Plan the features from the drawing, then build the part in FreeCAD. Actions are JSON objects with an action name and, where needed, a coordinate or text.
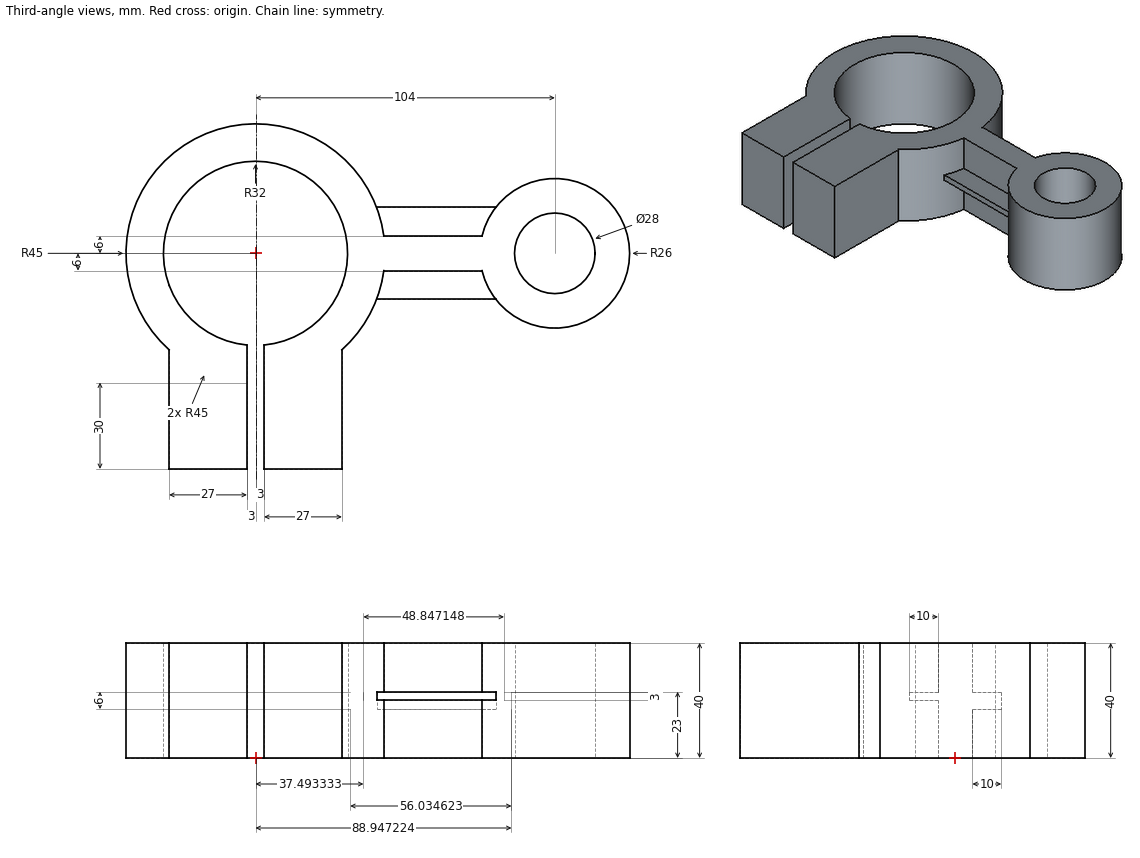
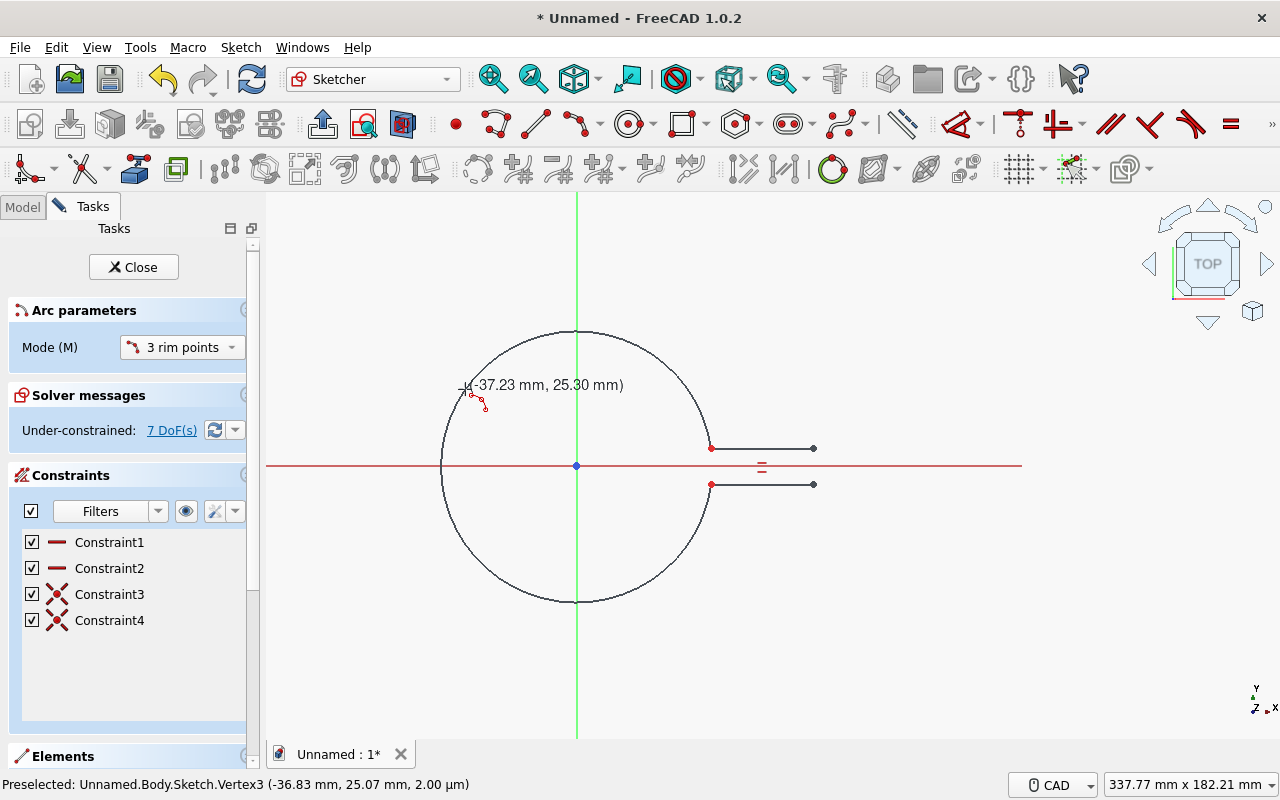
{"action": "left_click", "coordinate": [813, 485]}
{"action": "left_click", "coordinate": [813, 449]}
{"action": "left_click", "coordinate": [954, 509]}
{"action": "key", "text": "Escape"}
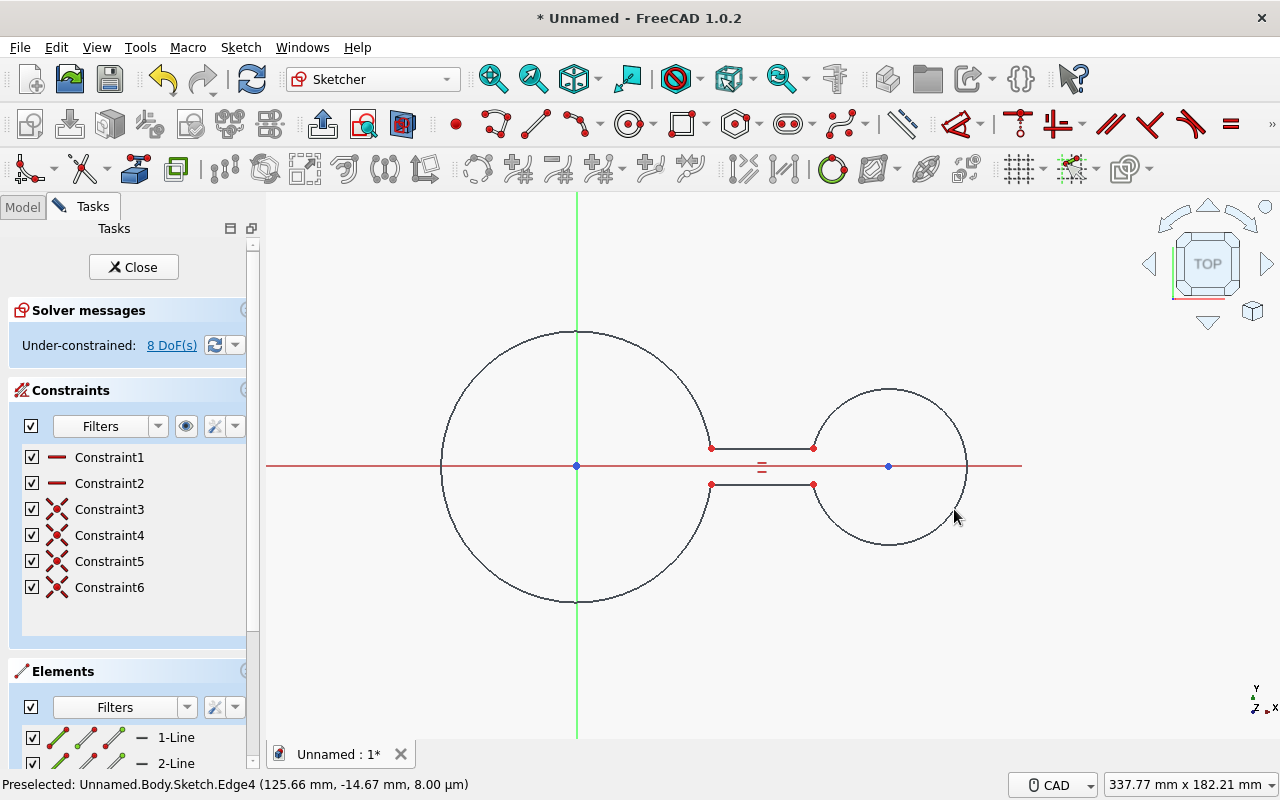
{"action": "left_click_drag", "start_coordinate": [567, 456], "coordinate": [587, 477]}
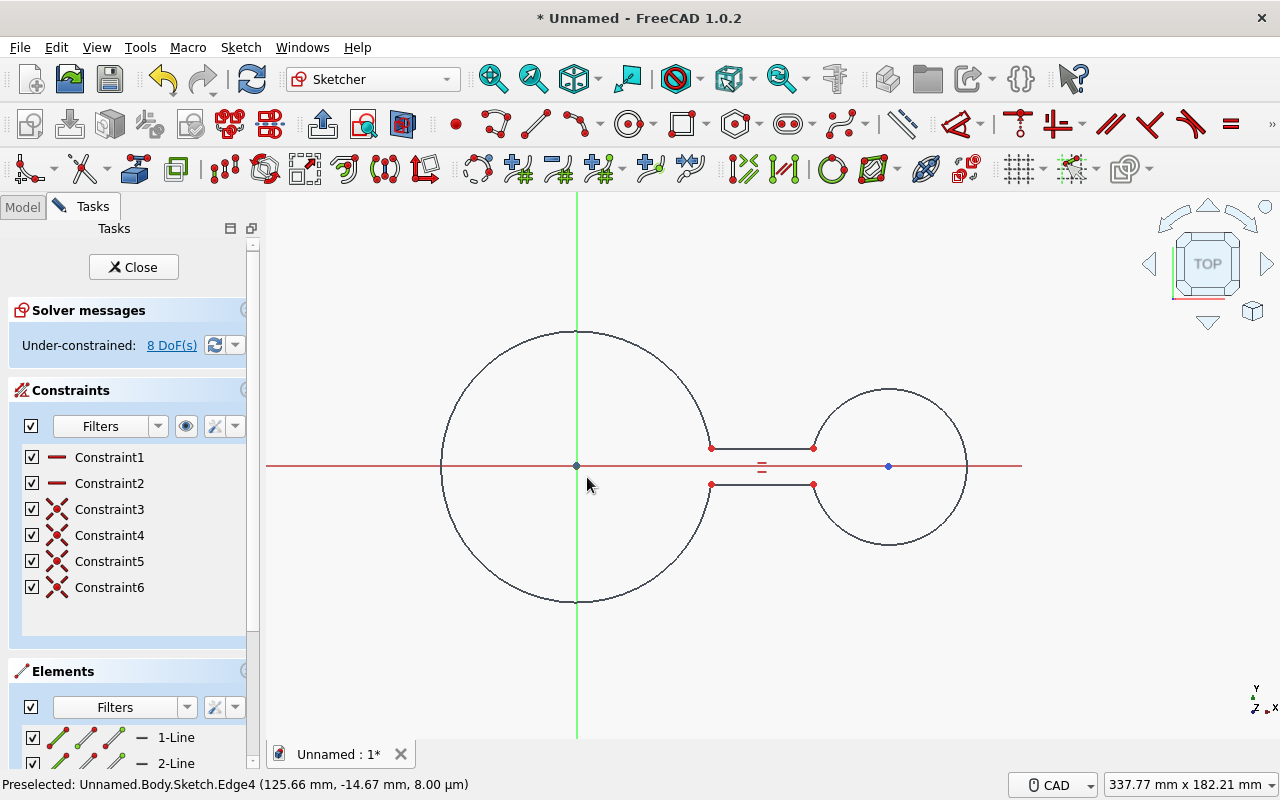
{"action": "left_click", "coordinate": [1018, 124]}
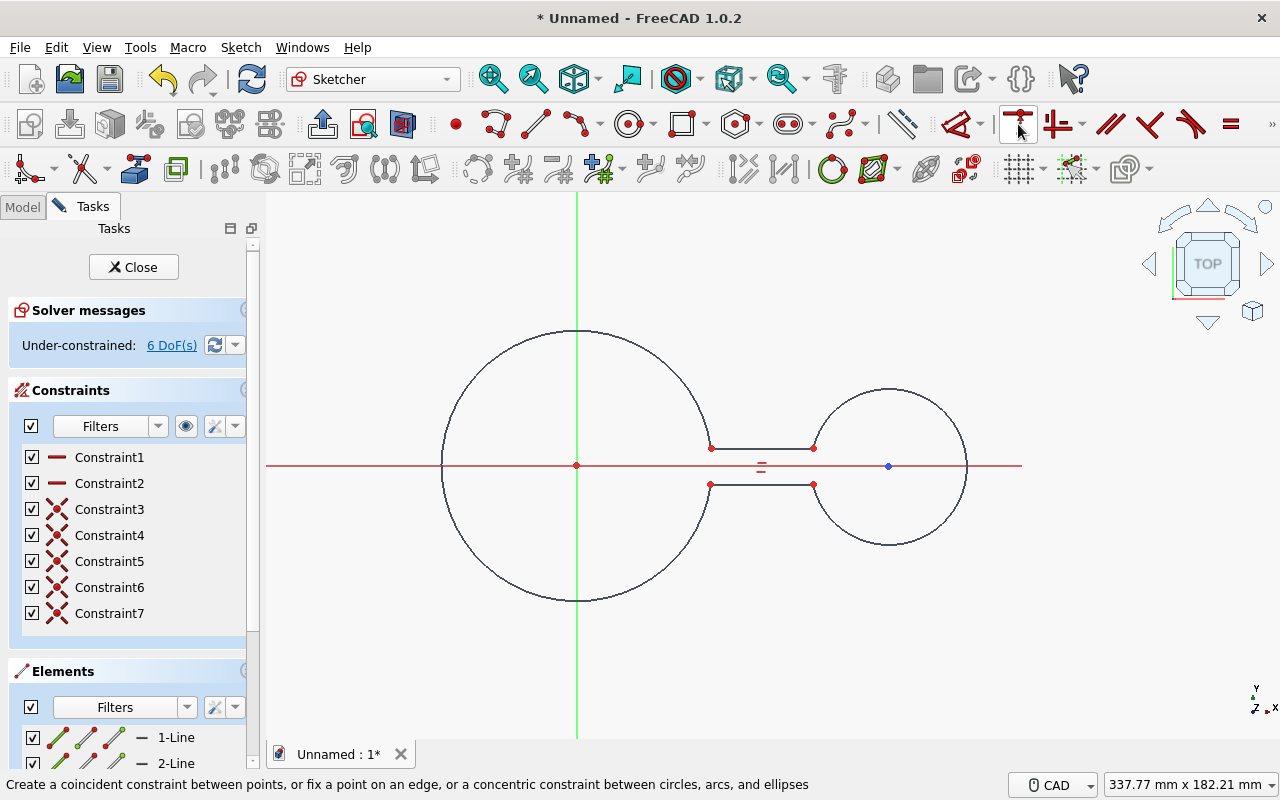
{"action": "left_click", "coordinate": [889, 467]}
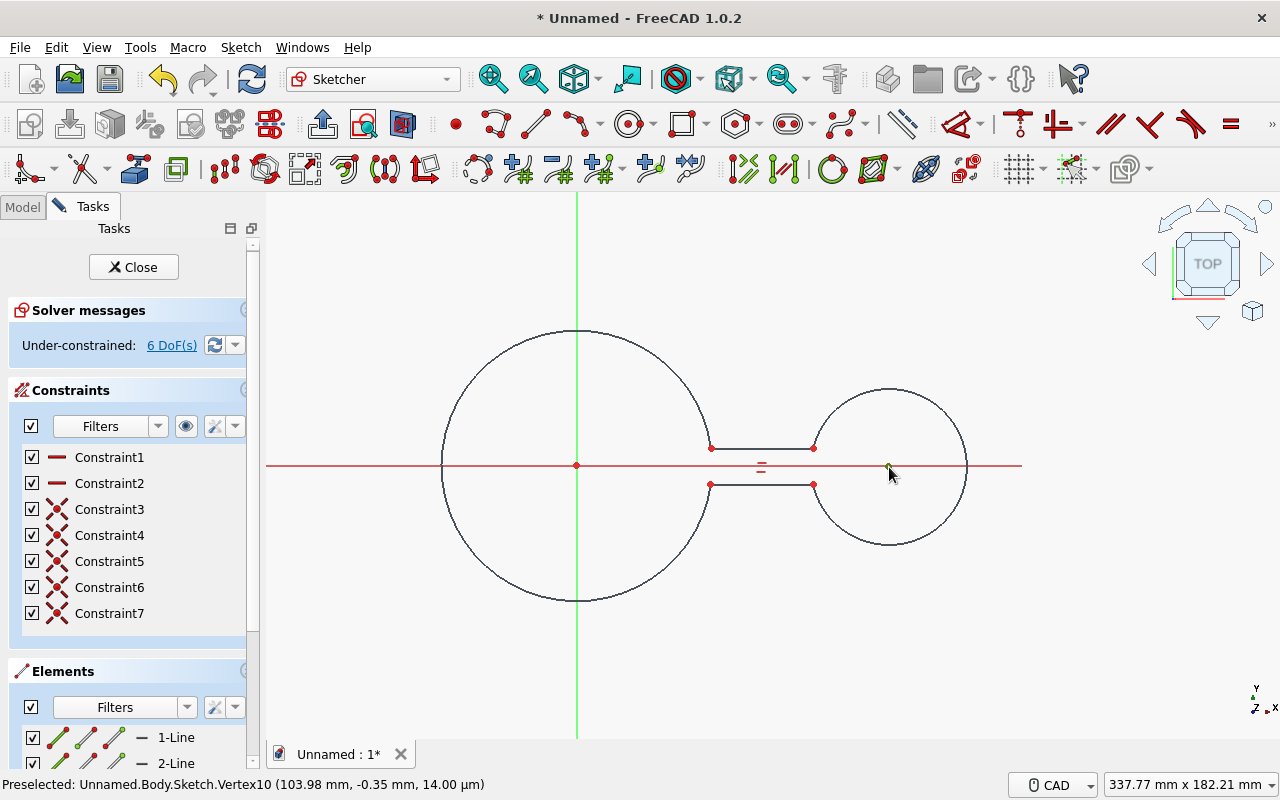
{"action": "left_click", "coordinate": [353, 466]}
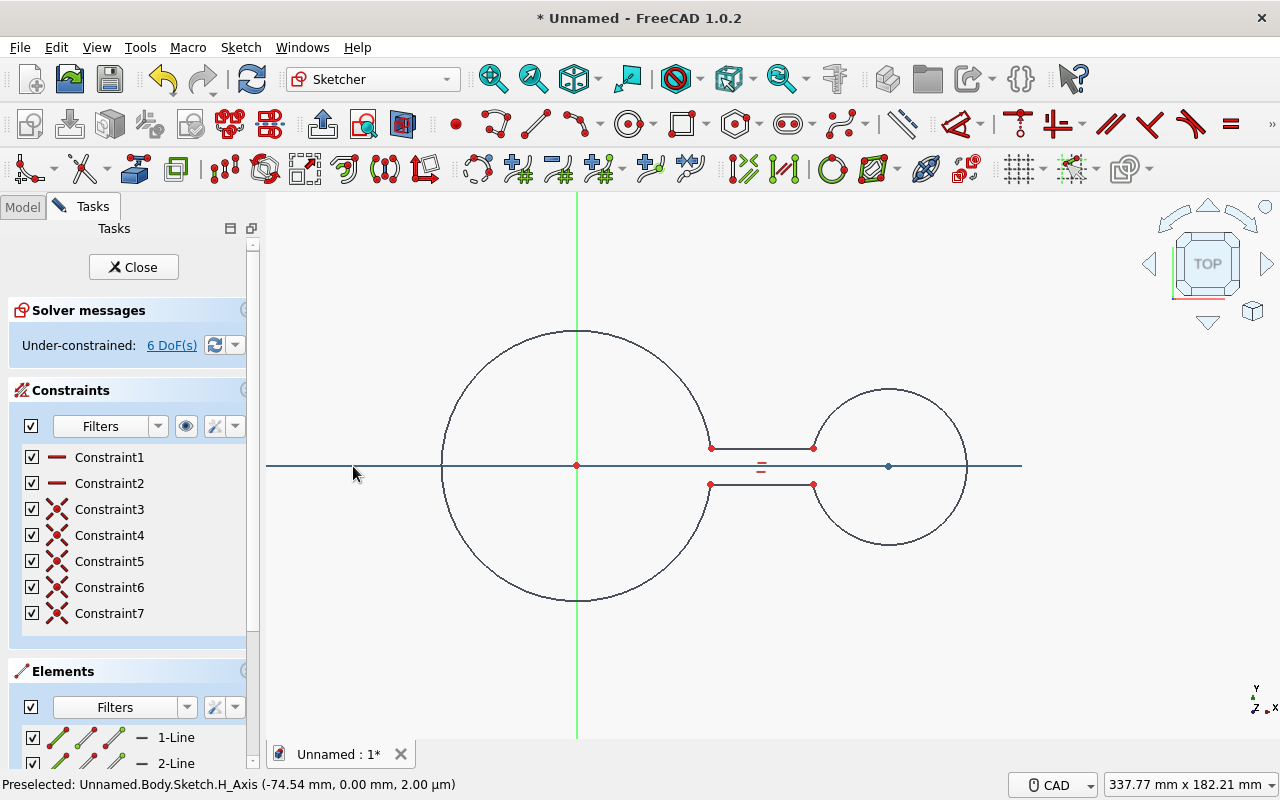
{"action": "left_click", "coordinate": [1018, 124]}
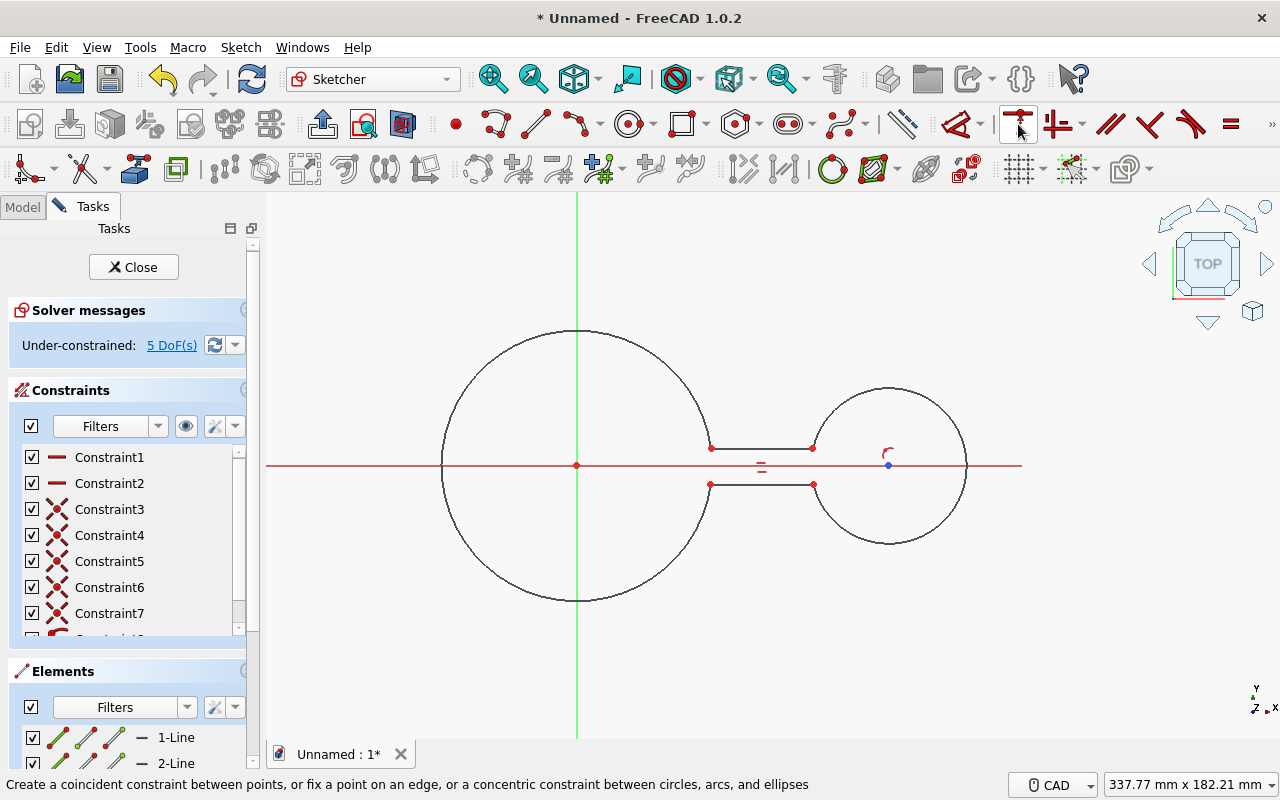
{"action": "key", "text": "d"}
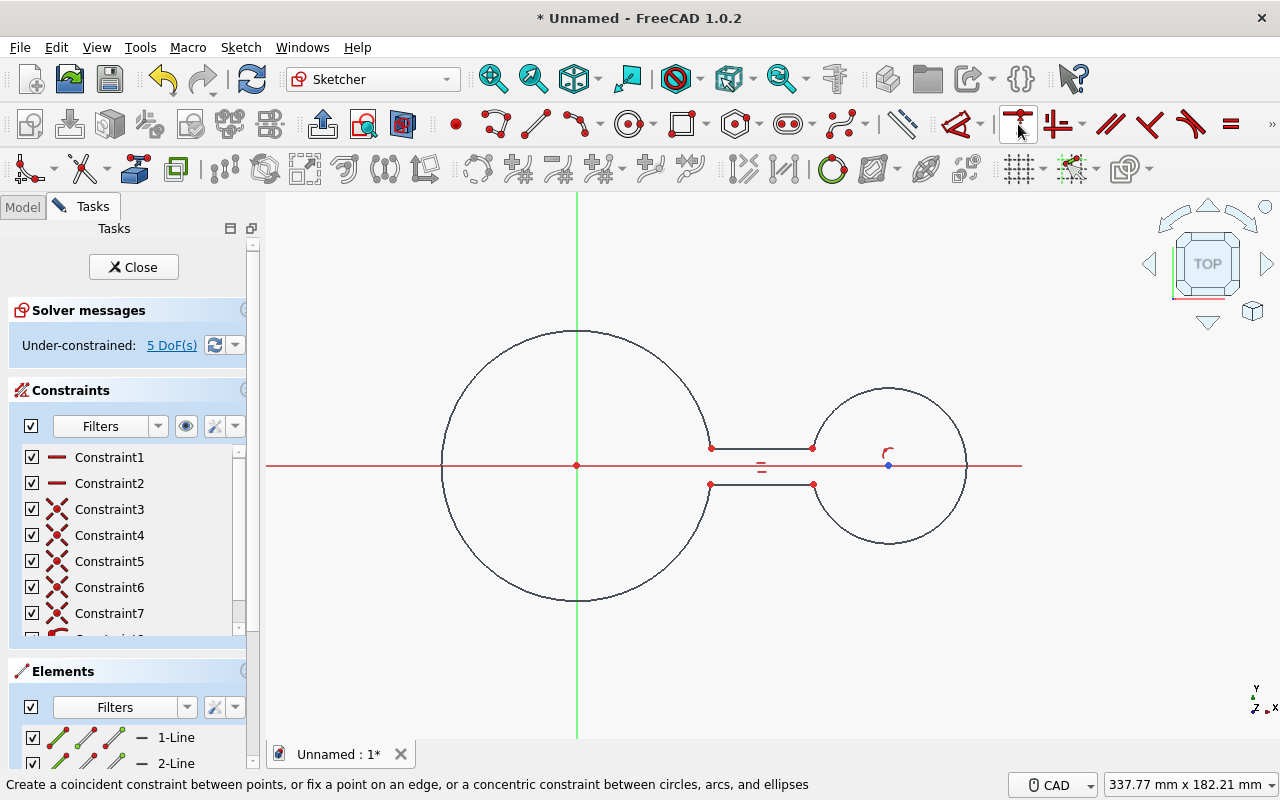
{"action": "left_click", "coordinate": [529, 339]}
{"action": "left_click", "coordinate": [518, 309]}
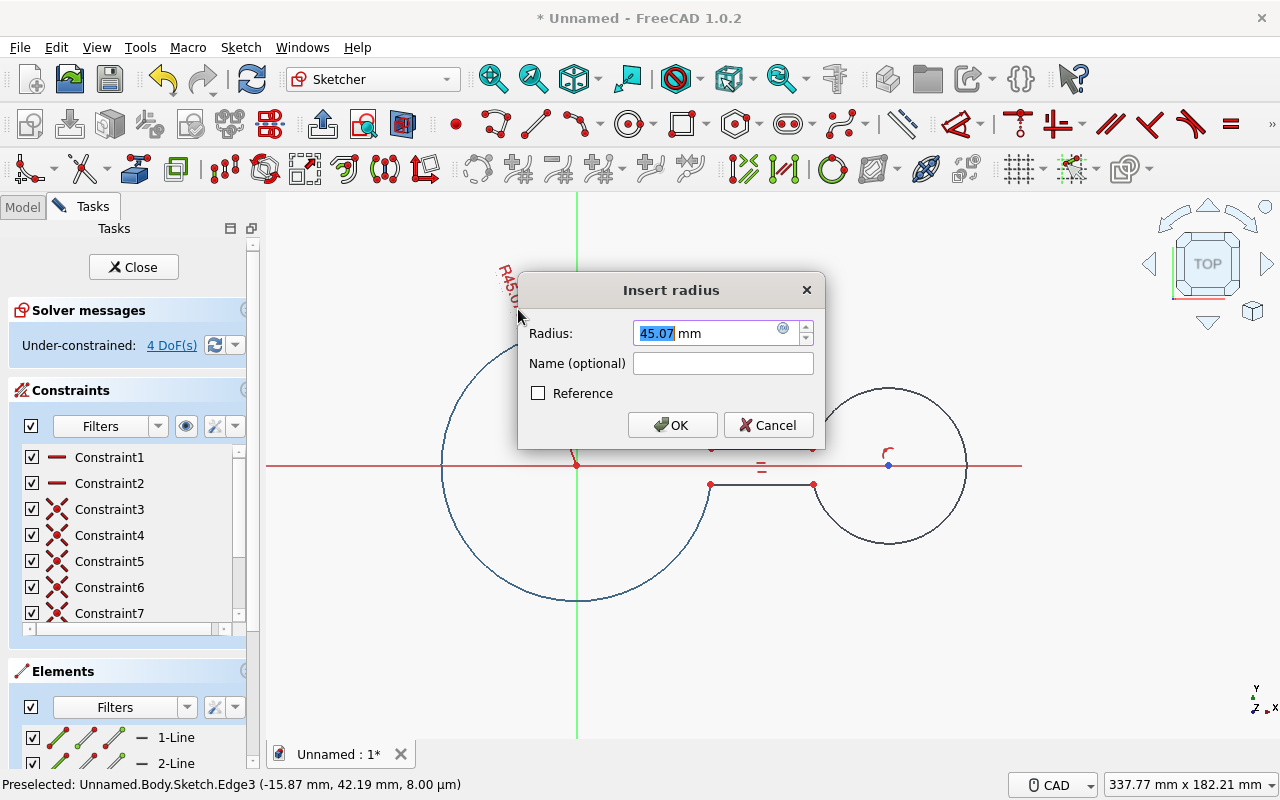
{"action": "type", "text": "45"}
{"action": "key", "text": "Return"}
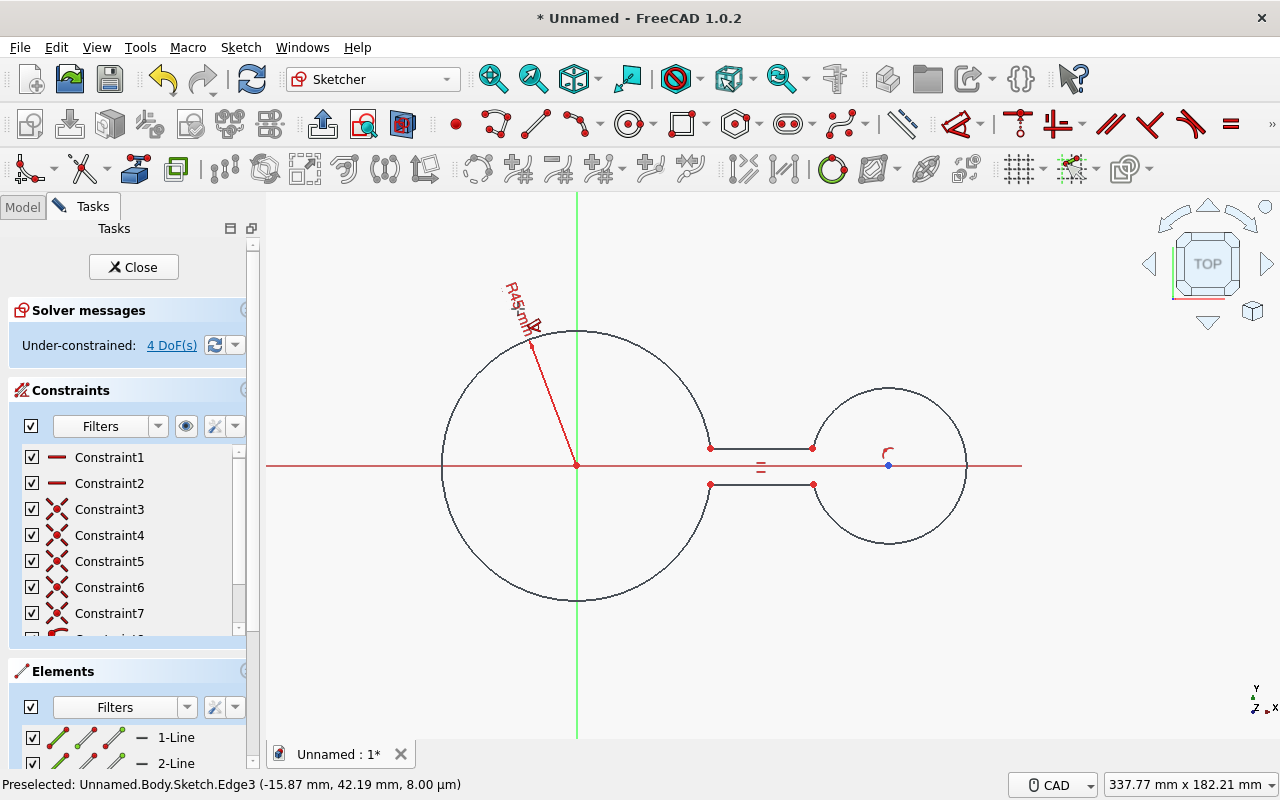
{"action": "left_click", "coordinate": [921, 537]}
{"action": "left_click", "coordinate": [934, 566]}